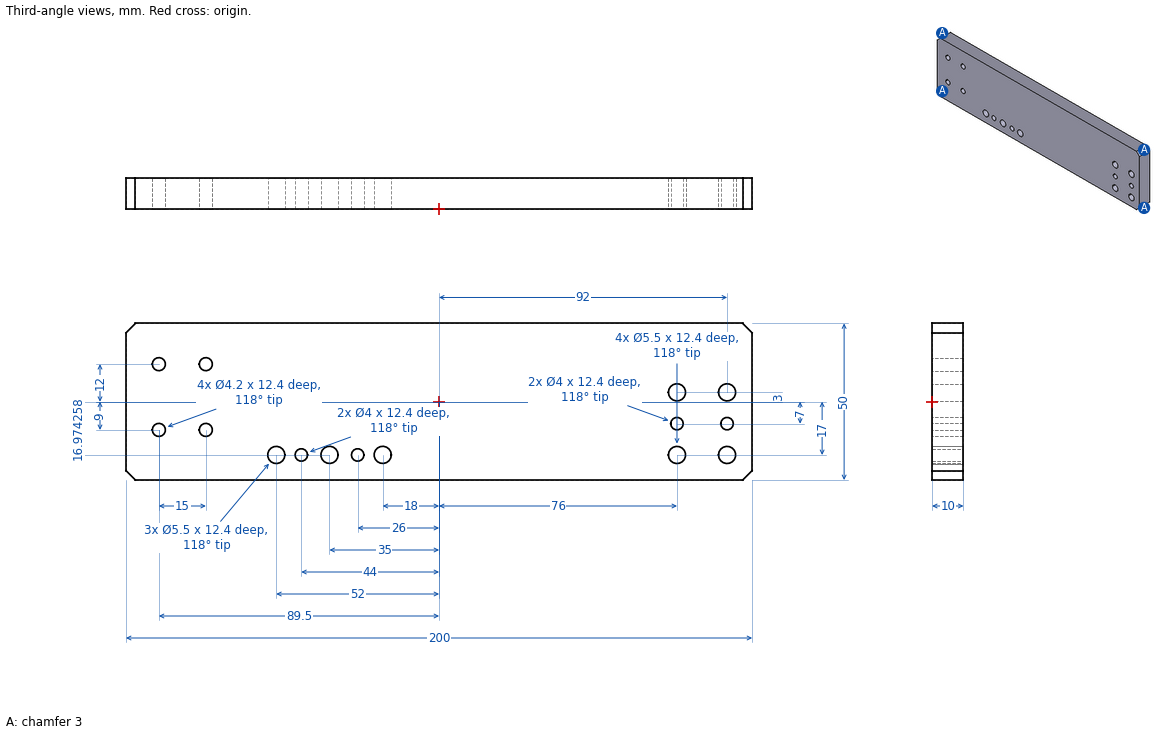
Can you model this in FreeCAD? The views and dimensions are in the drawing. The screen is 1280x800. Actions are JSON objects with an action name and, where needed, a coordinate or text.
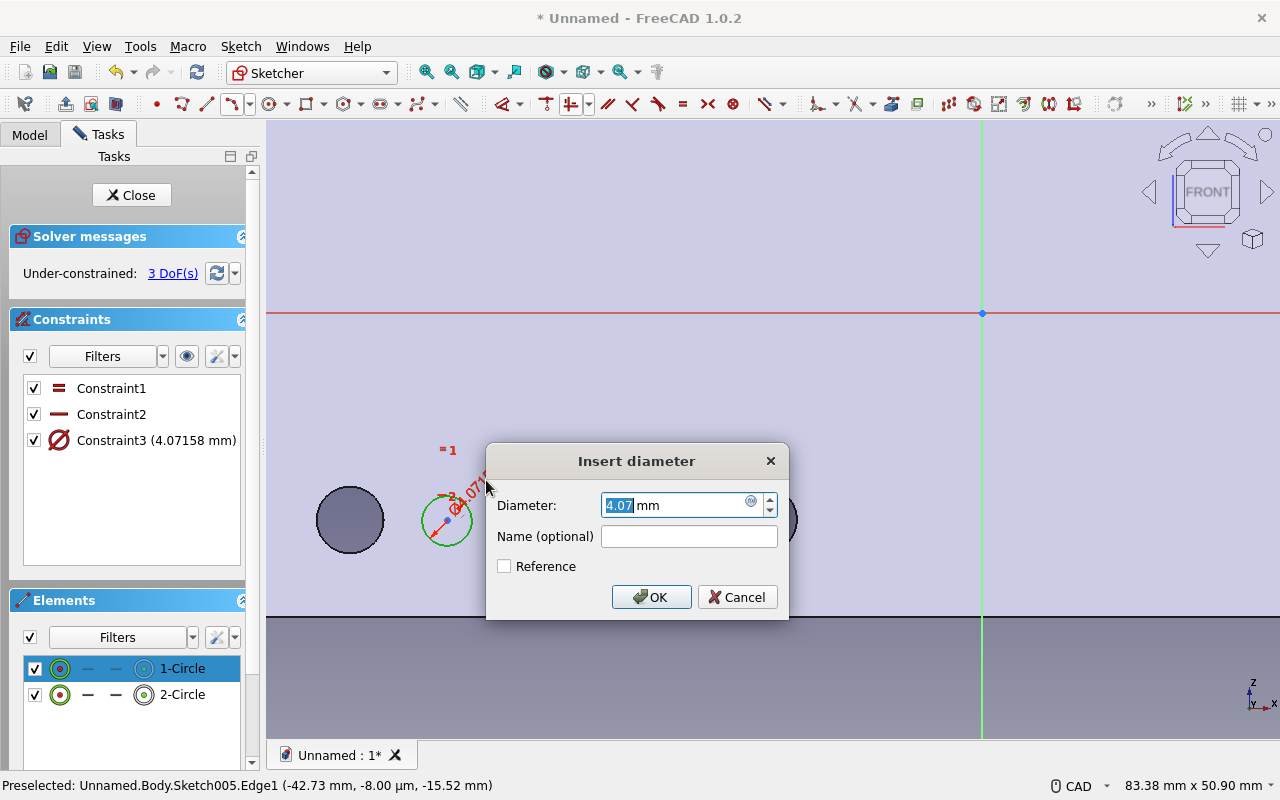
{"action": "type", "text": "4"}
{"action": "key", "text": "Return"}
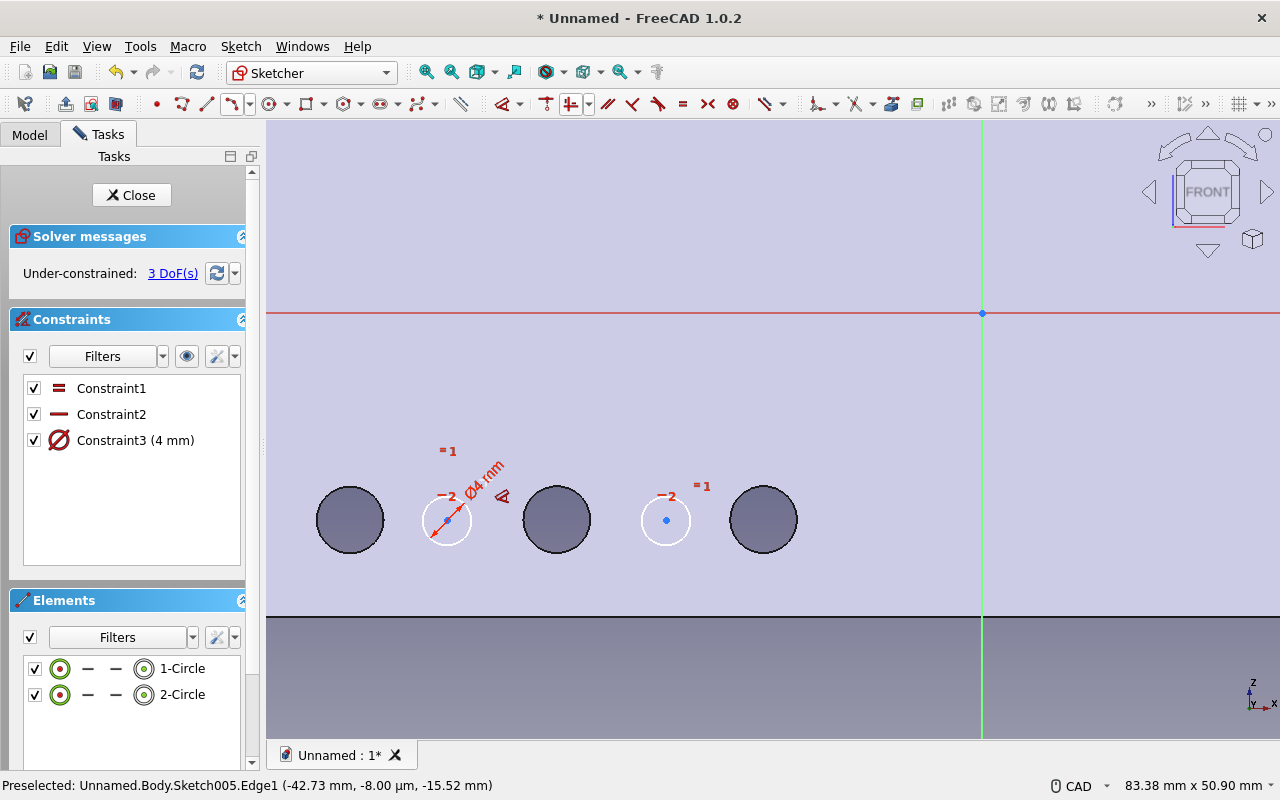
{"action": "left_click", "coordinate": [447, 521]}
{"action": "left_click", "coordinate": [715, 279]}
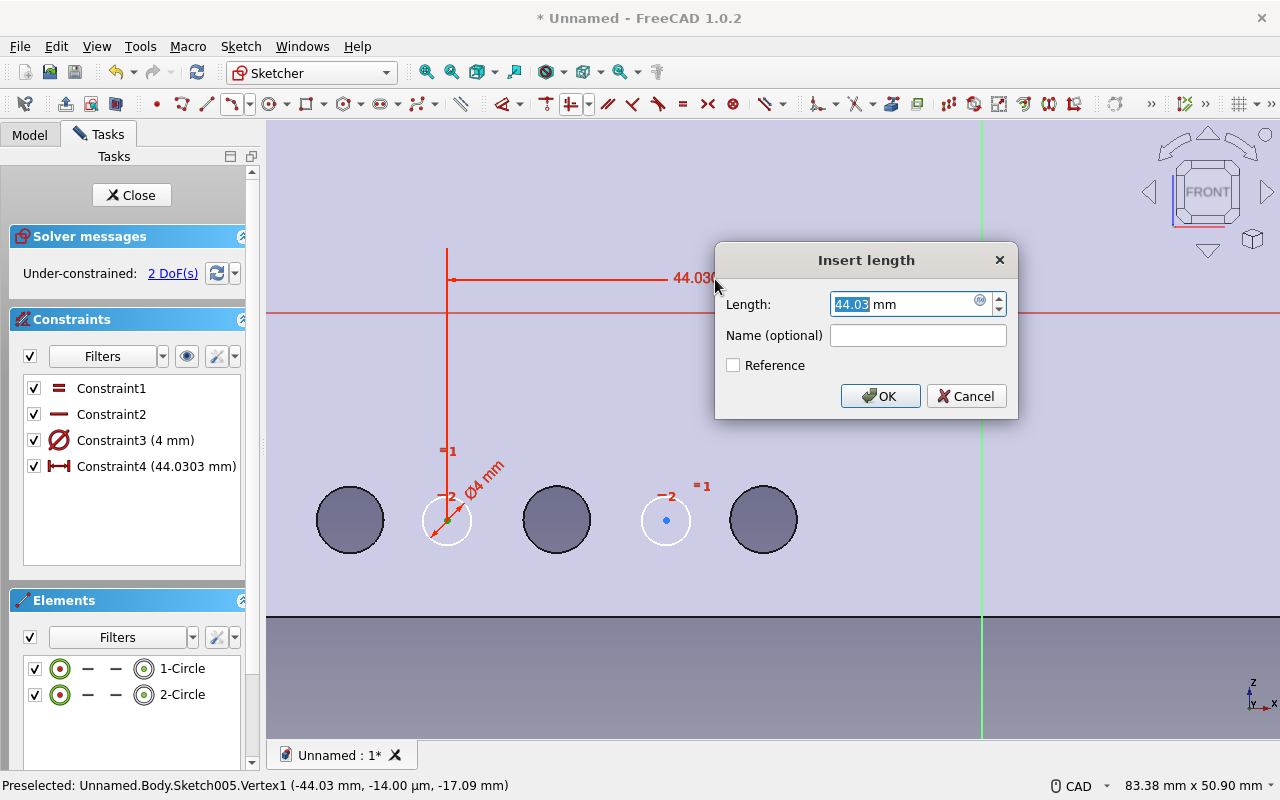
{"action": "type", "text": "44"}
{"action": "key", "text": "Return"}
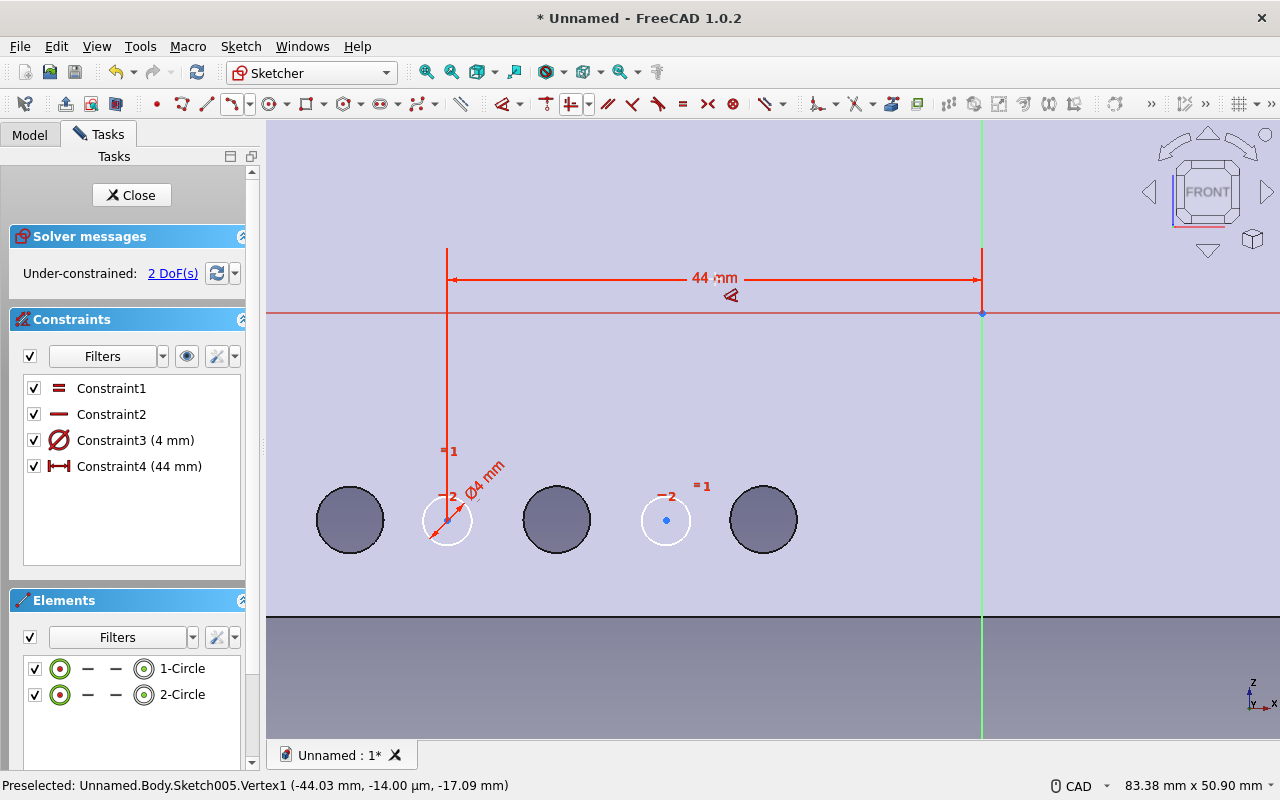
{"action": "left_click", "coordinate": [447, 521]}
{"action": "left_click", "coordinate": [1016, 417]}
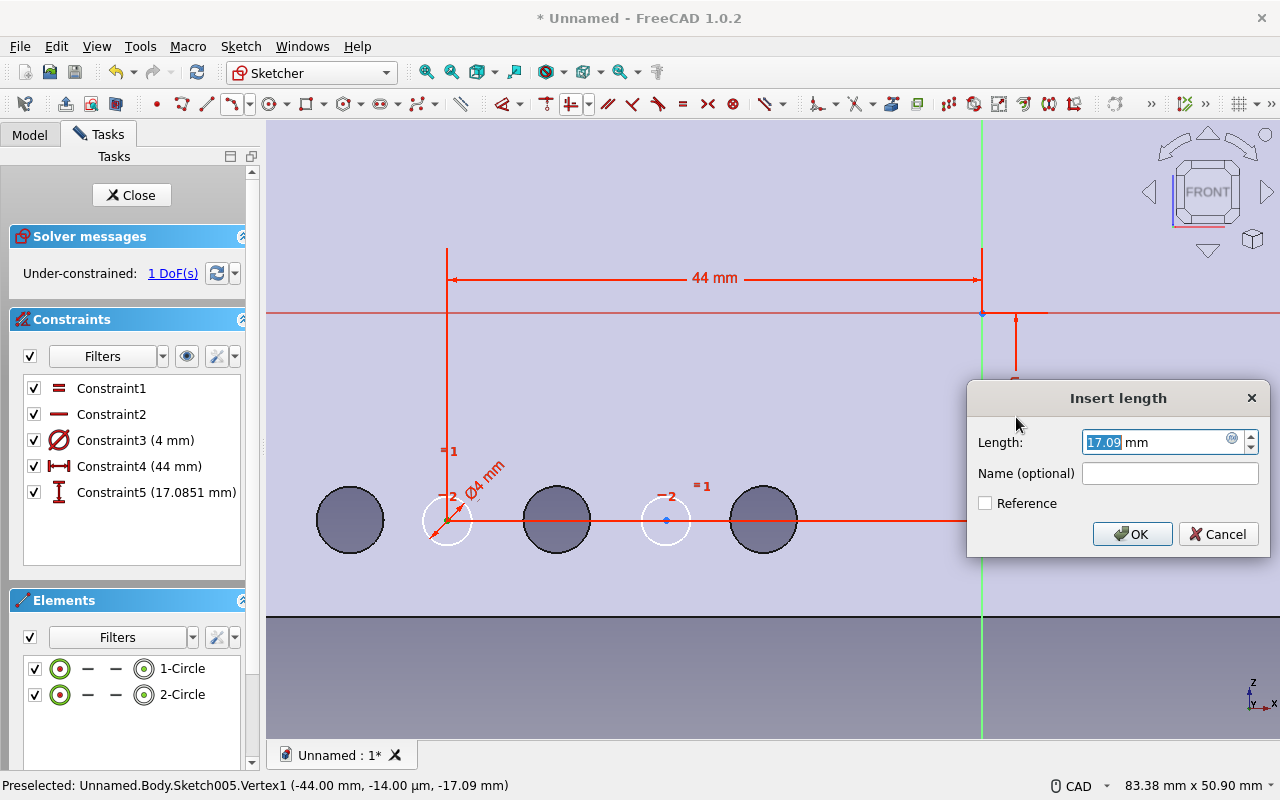
{"action": "type", "text": "17"}
{"action": "key", "text": "Return"}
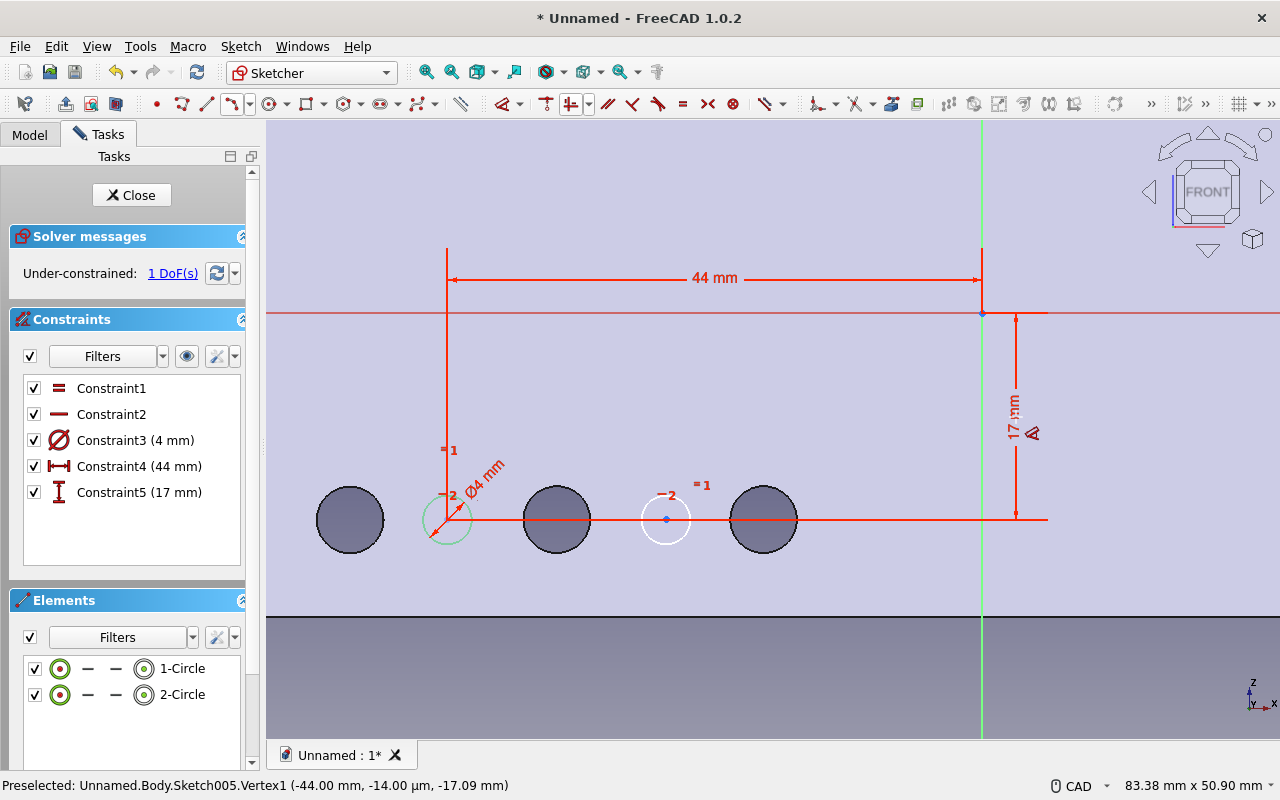
{"action": "left_click", "coordinate": [666, 520]}
{"action": "left_click", "coordinate": [824, 279]}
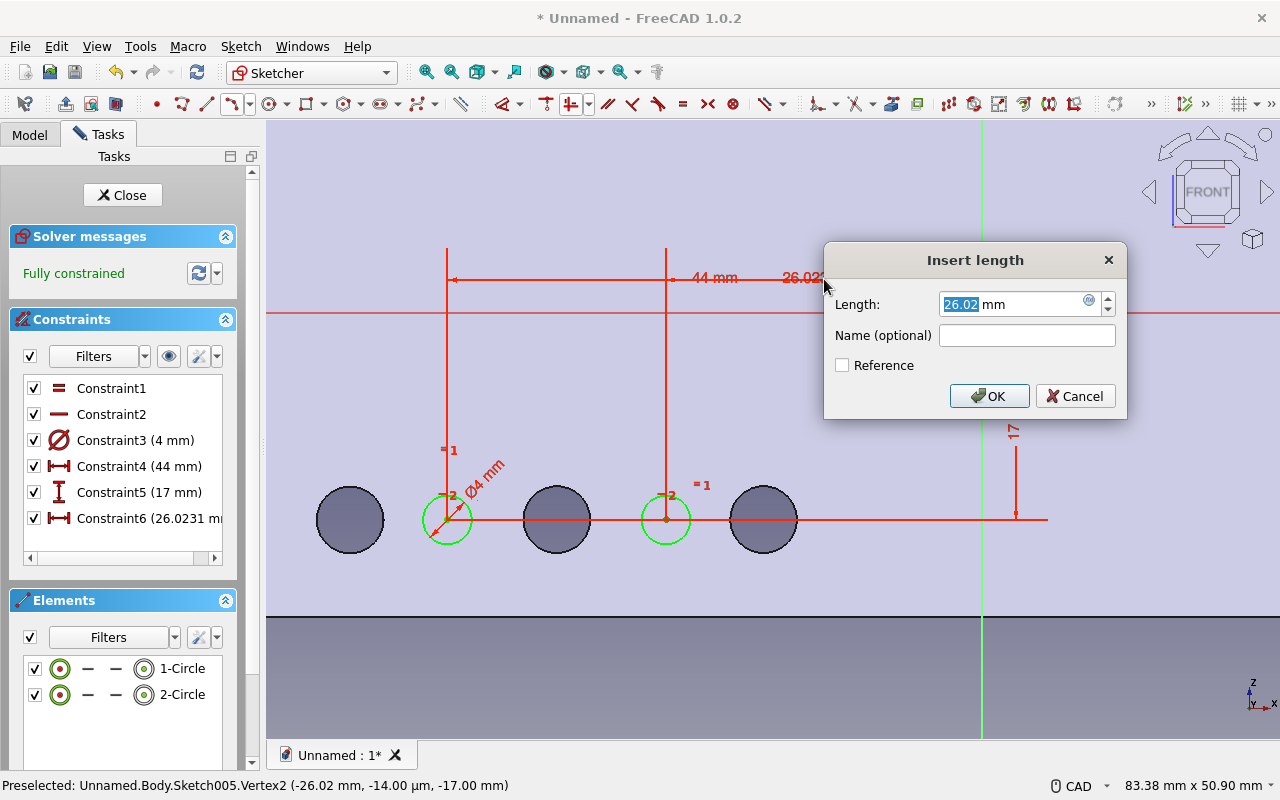
{"action": "type", "text": "26"}
{"action": "key", "text": "Return"}
{"action": "key", "text": "Escape"}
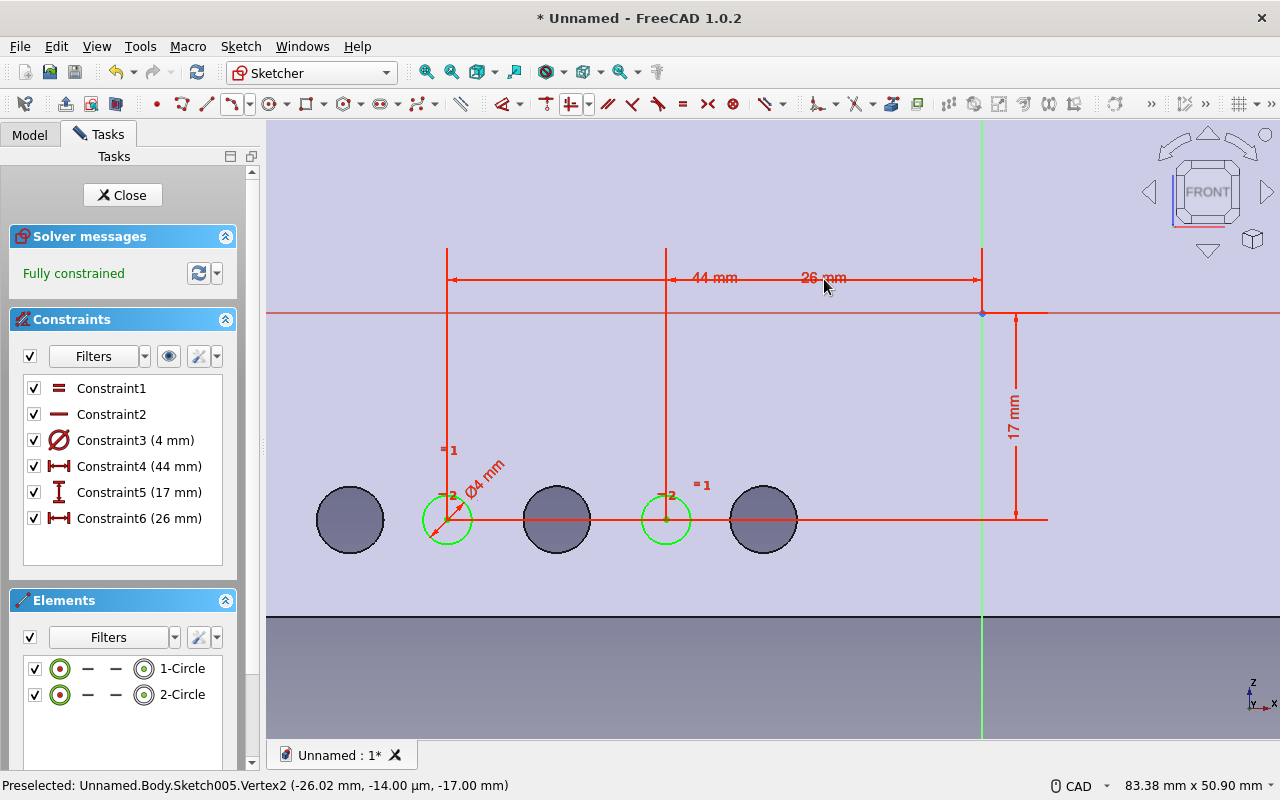
{"action": "left_click", "coordinate": [123, 195]}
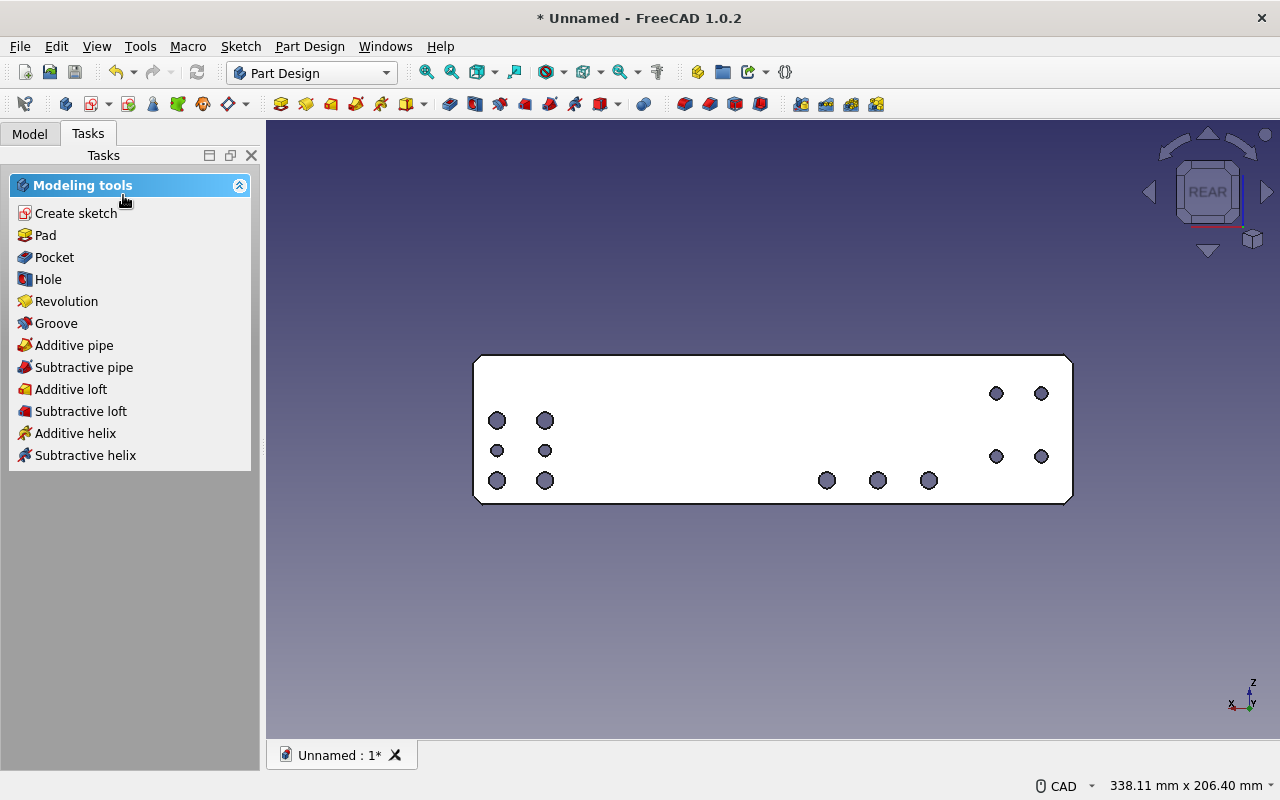
{"action": "left_click", "coordinate": [475, 104]}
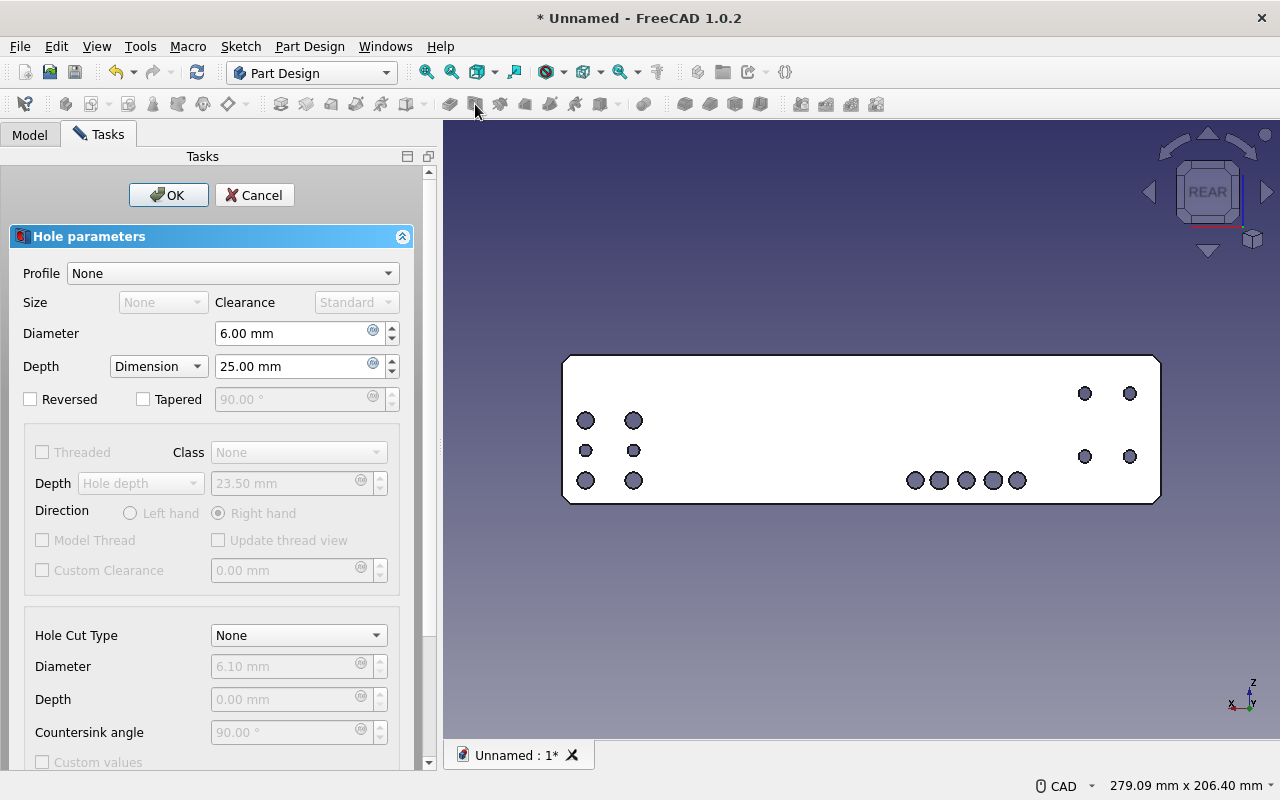
{"action": "triple_click", "coordinate": [300, 334]}